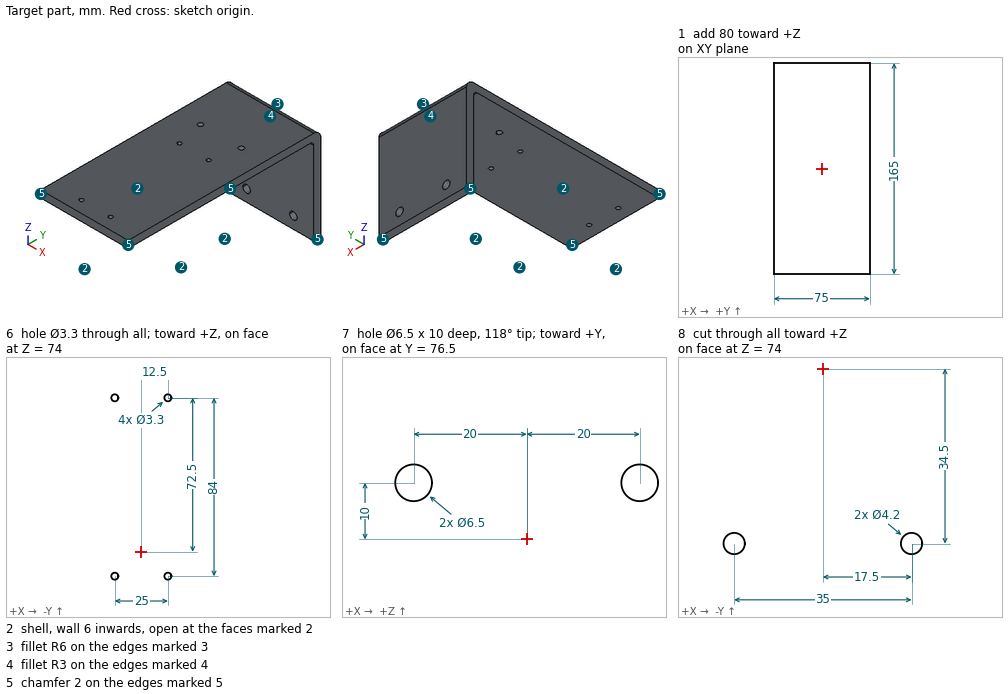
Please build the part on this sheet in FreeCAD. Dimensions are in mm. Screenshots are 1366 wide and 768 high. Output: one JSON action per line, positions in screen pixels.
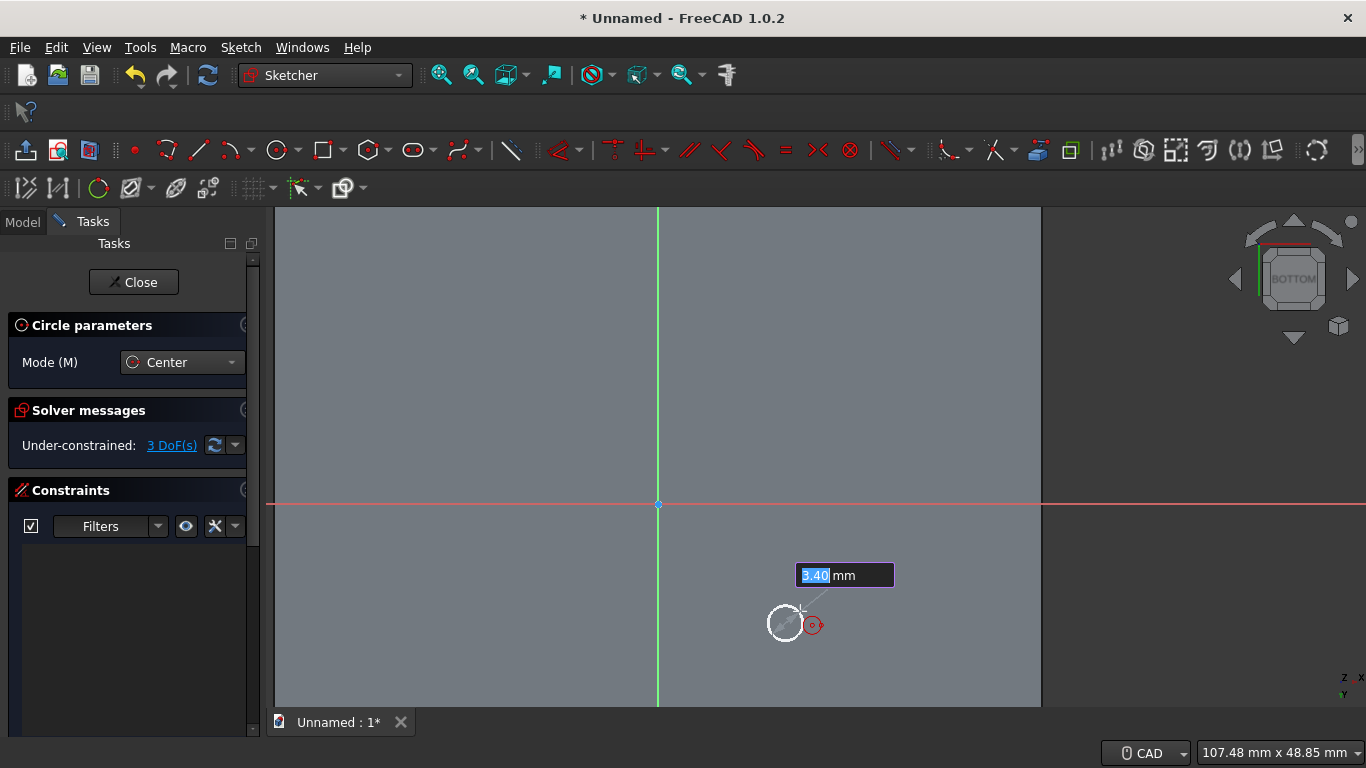
{"action": "left_click", "coordinate": [798, 610]}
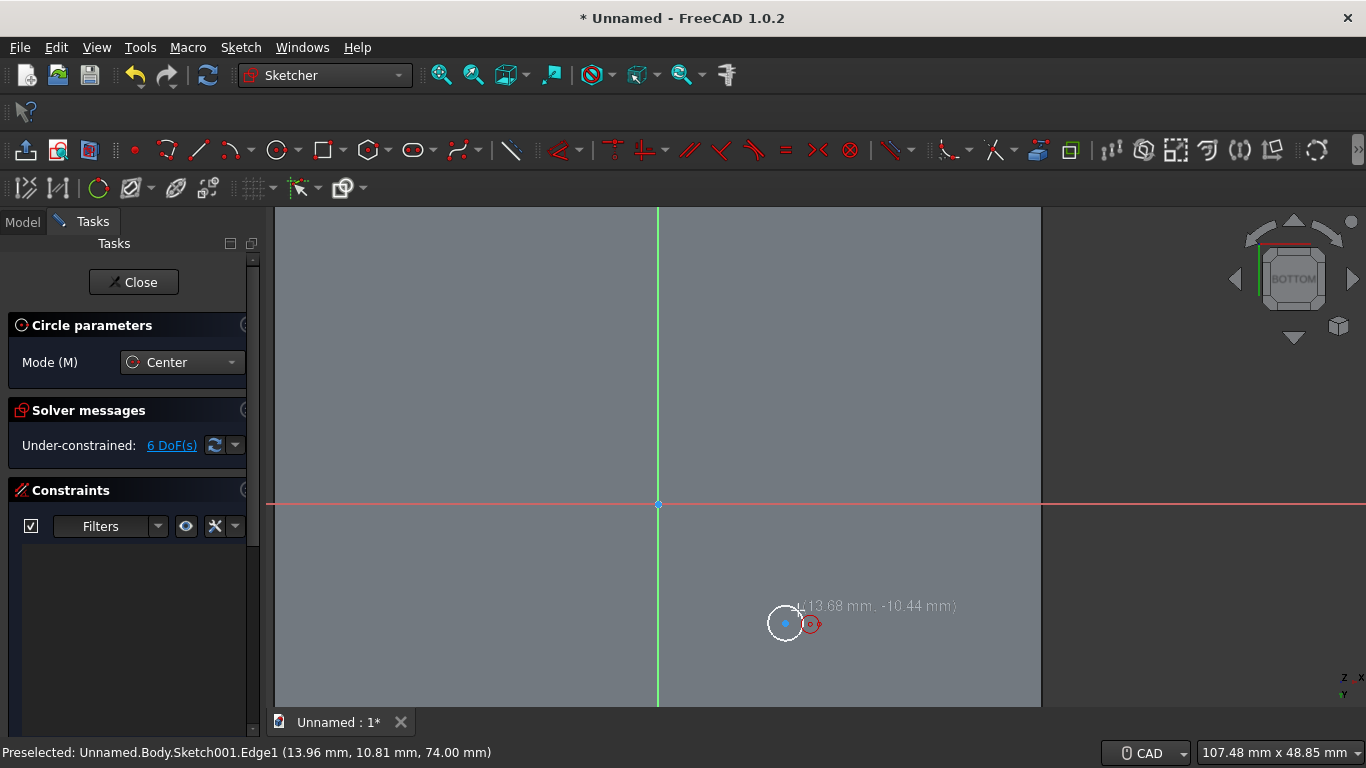
{"action": "scroll", "coordinate": [530, 622], "scroll_direction": "up", "scroll_amount": 2}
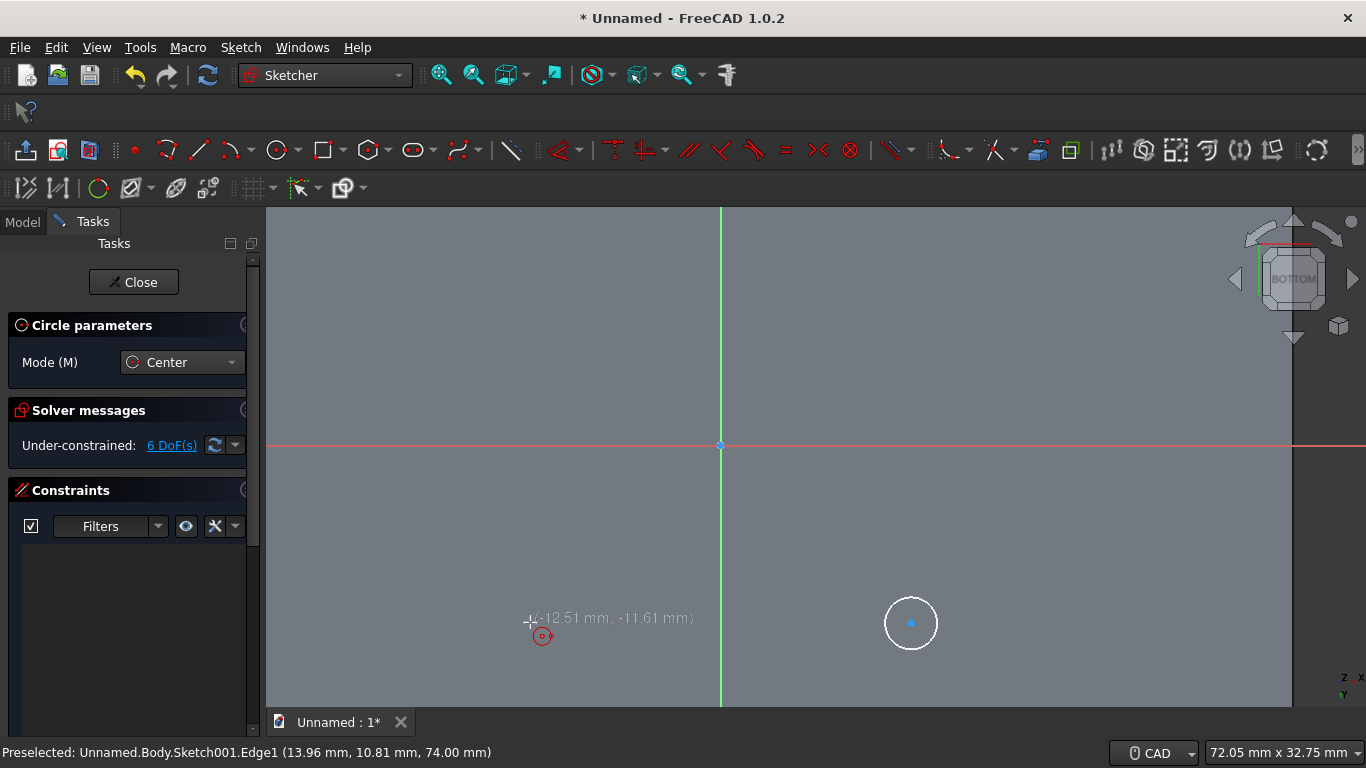
{"action": "scroll", "coordinate": [756, 613], "scroll_direction": "down", "scroll_amount": 7}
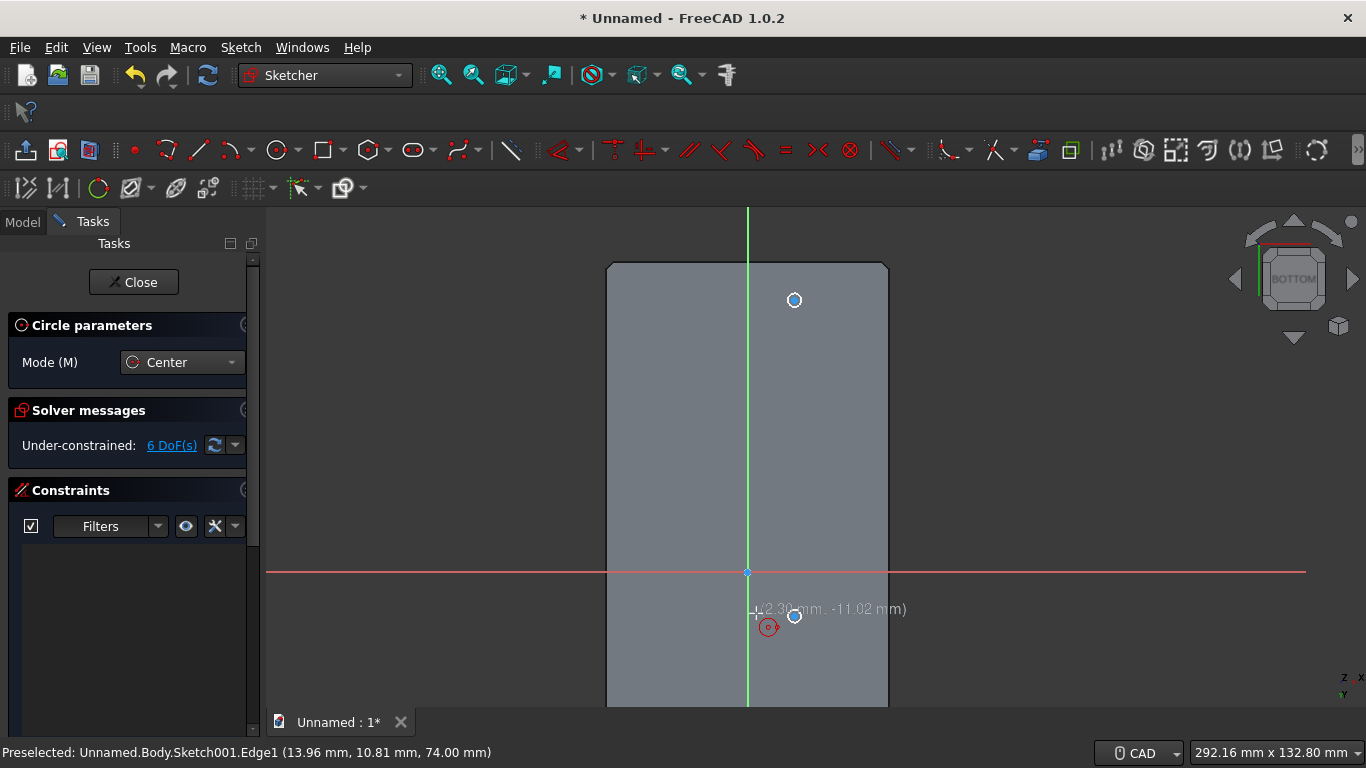
{"action": "left_click", "coordinate": [701, 616]}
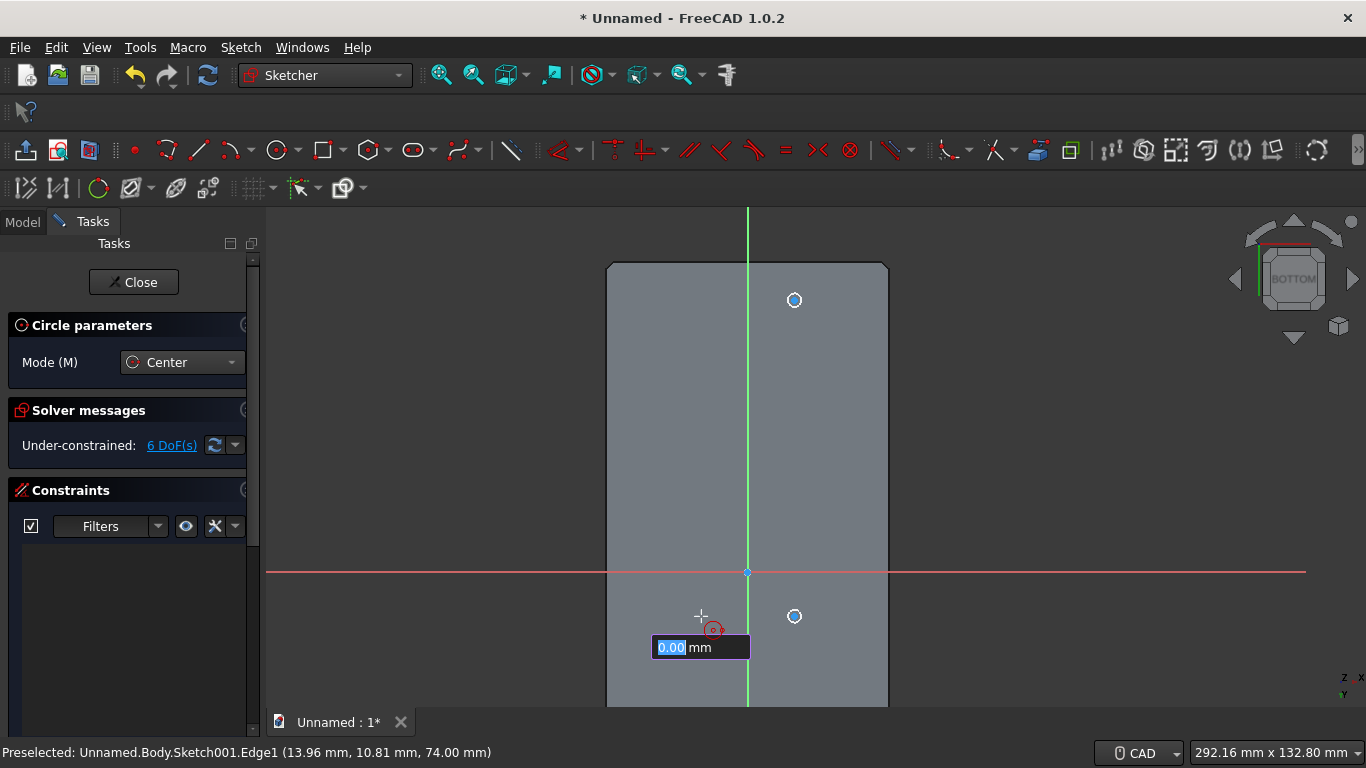
{"action": "scroll", "coordinate": [705, 611], "scroll_direction": "up", "scroll_amount": 5}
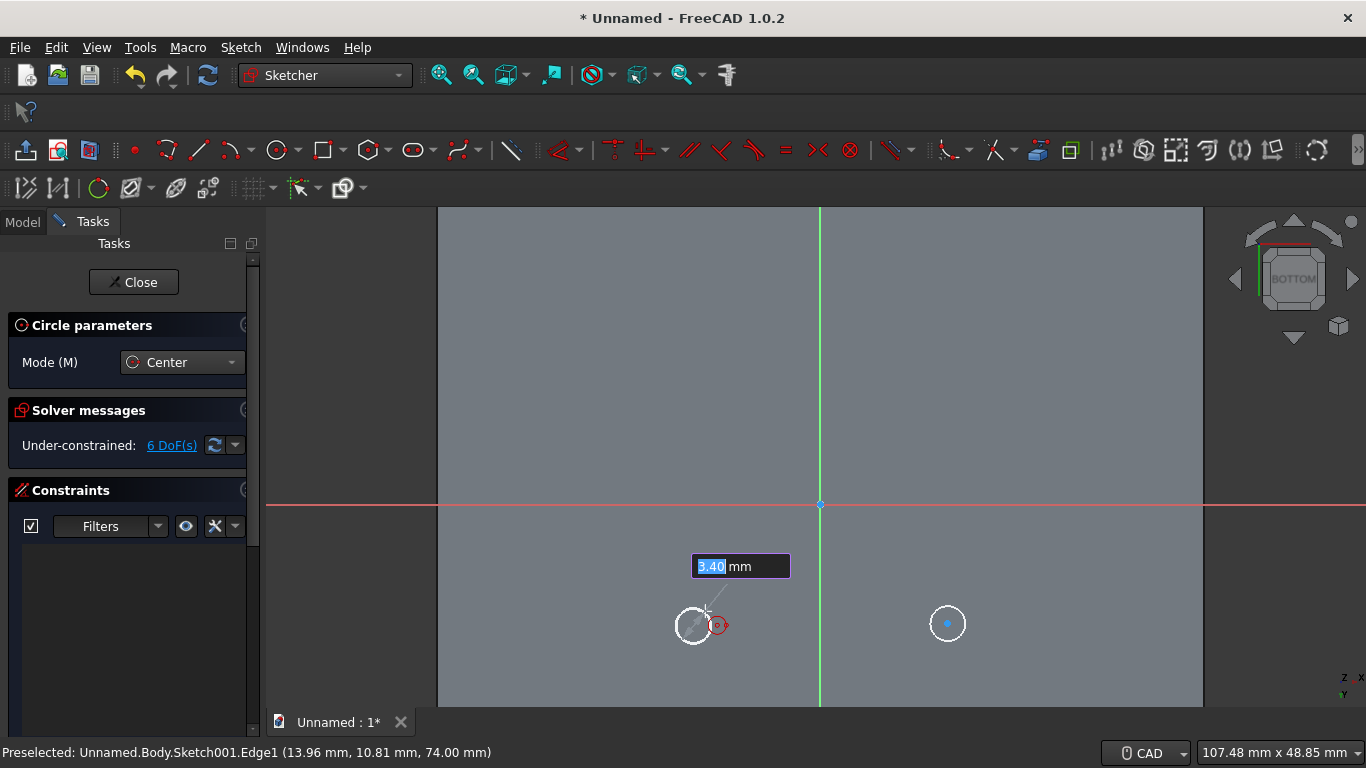
{"action": "left_click", "coordinate": [704, 610]}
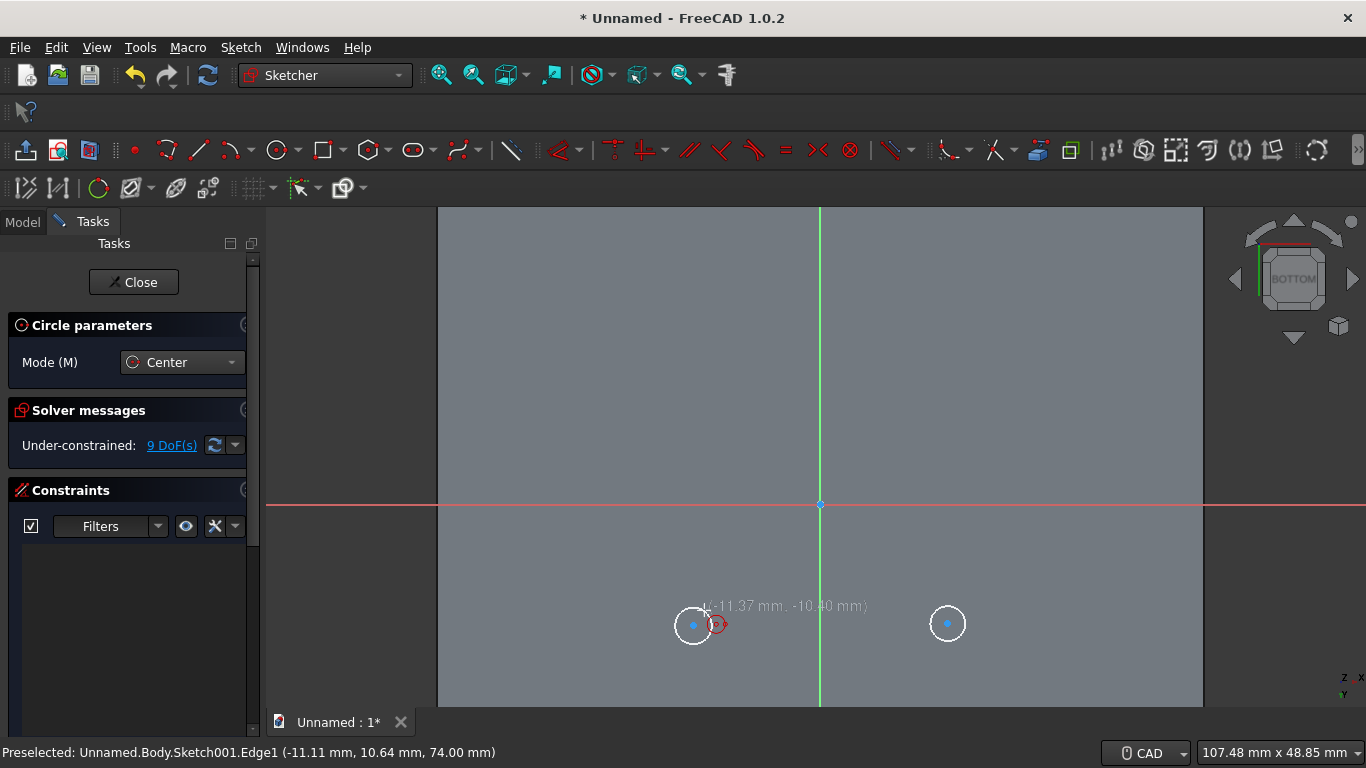
{"action": "scroll", "coordinate": [705, 611], "scroll_direction": "down", "scroll_amount": 5}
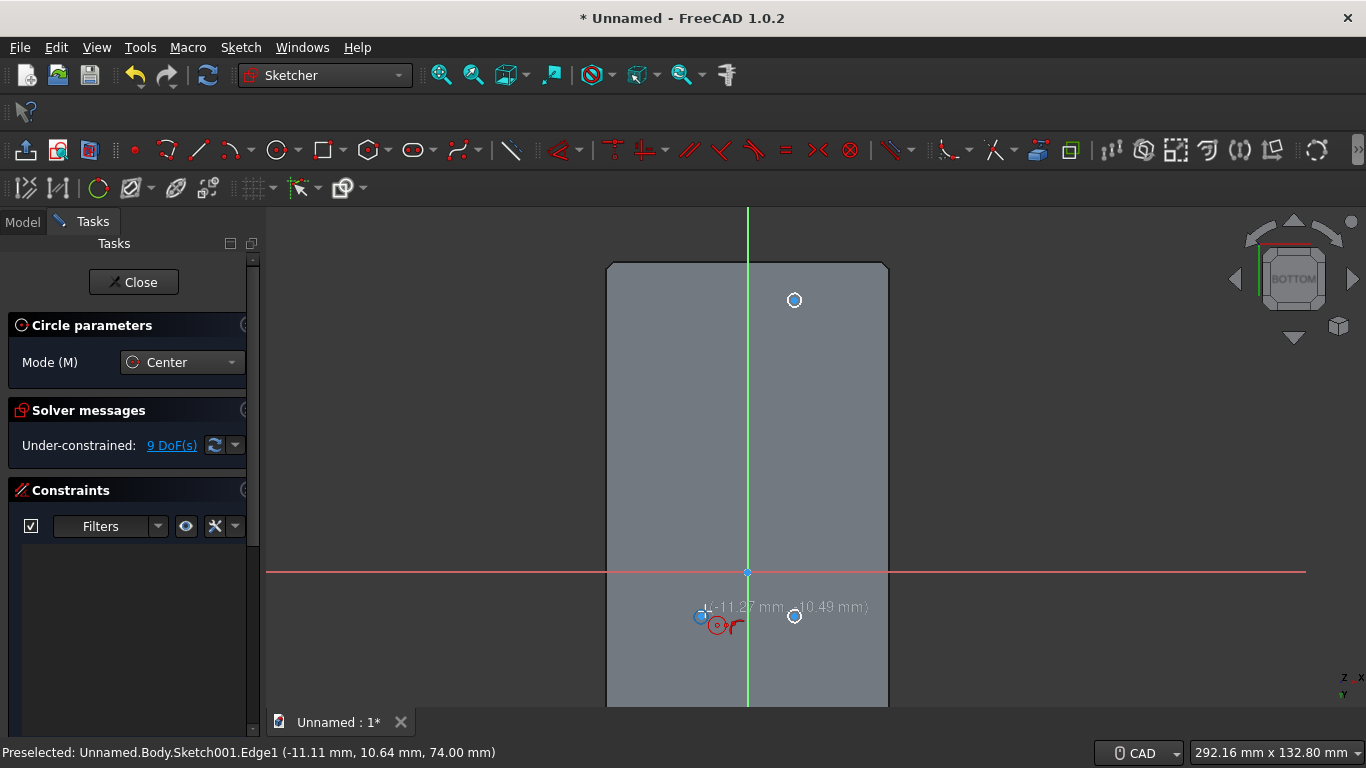
{"action": "scroll", "coordinate": [701, 299], "scroll_direction": "up", "scroll_amount": 7}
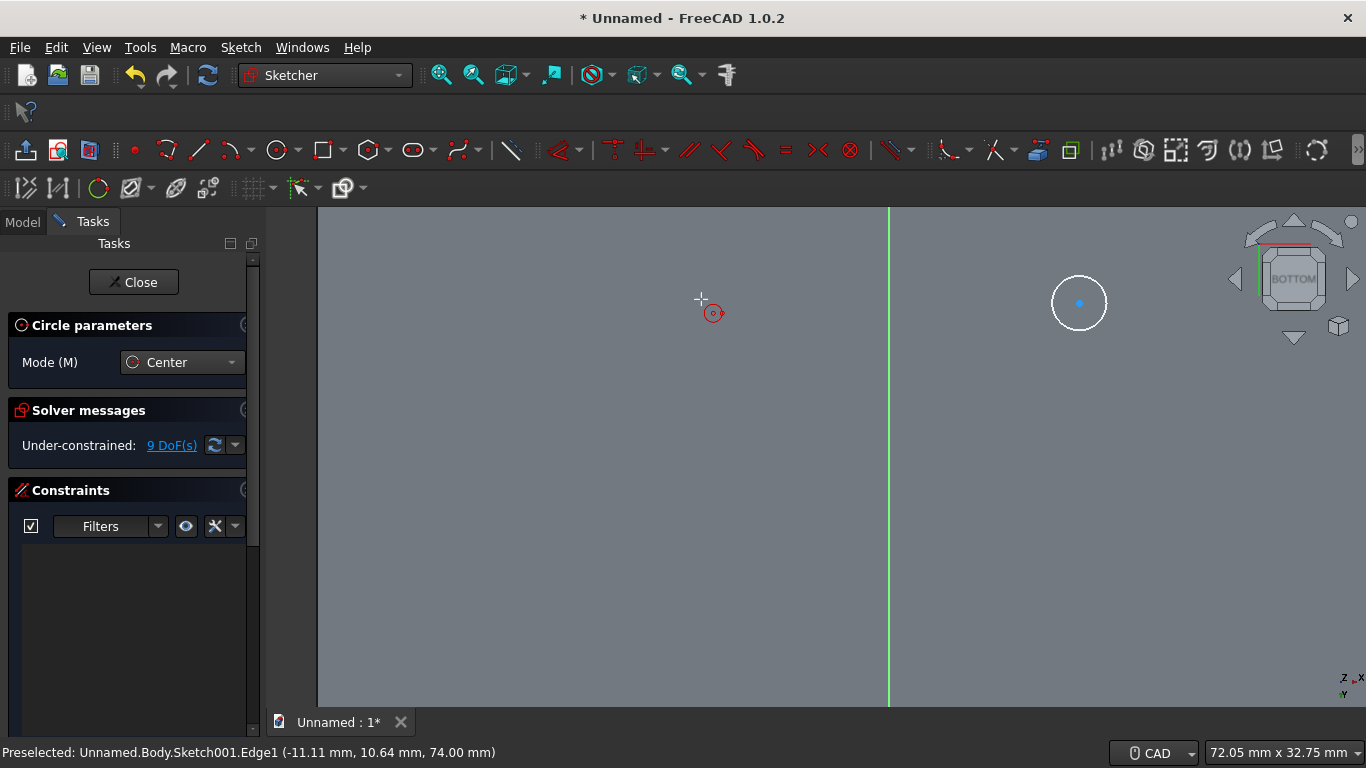
{"action": "scroll", "coordinate": [701, 298], "scroll_direction": "down", "scroll_amount": 7}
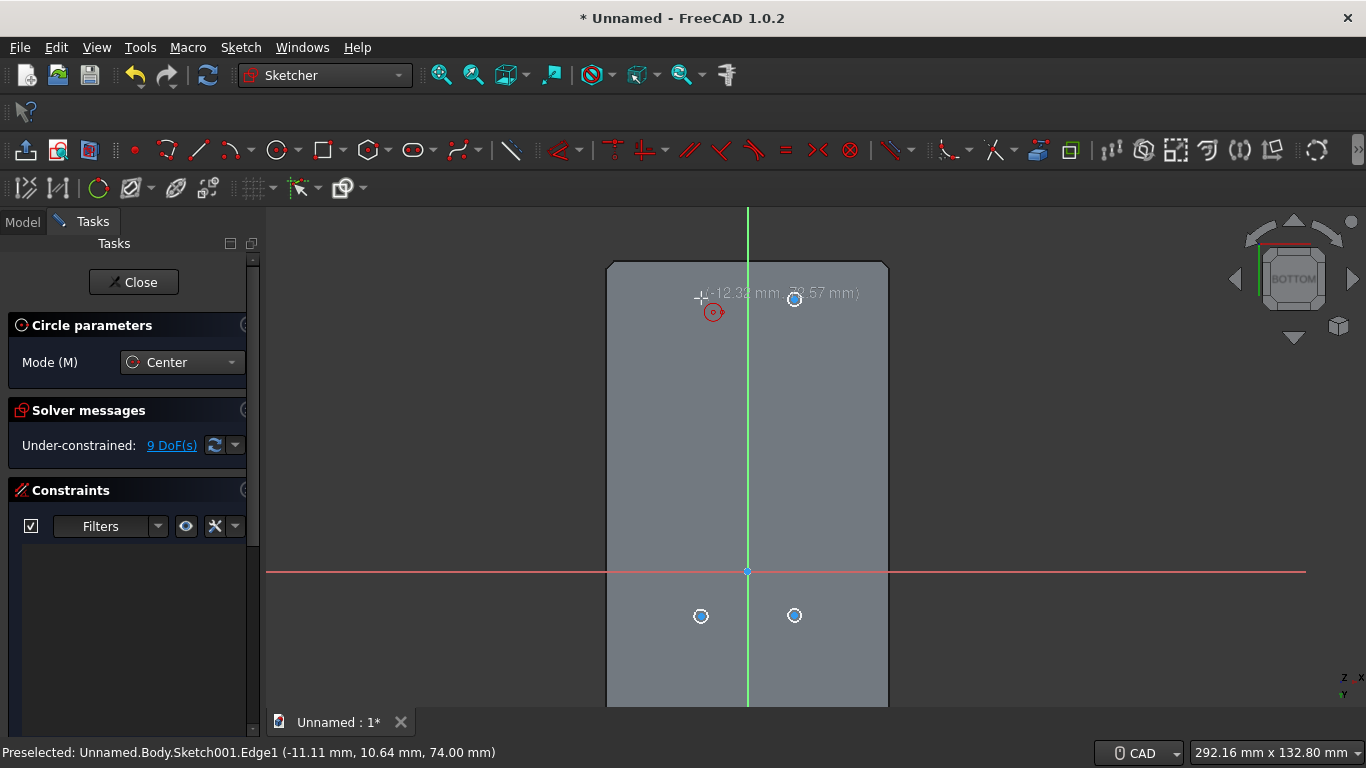
{"action": "left_click", "coordinate": [701, 299]}